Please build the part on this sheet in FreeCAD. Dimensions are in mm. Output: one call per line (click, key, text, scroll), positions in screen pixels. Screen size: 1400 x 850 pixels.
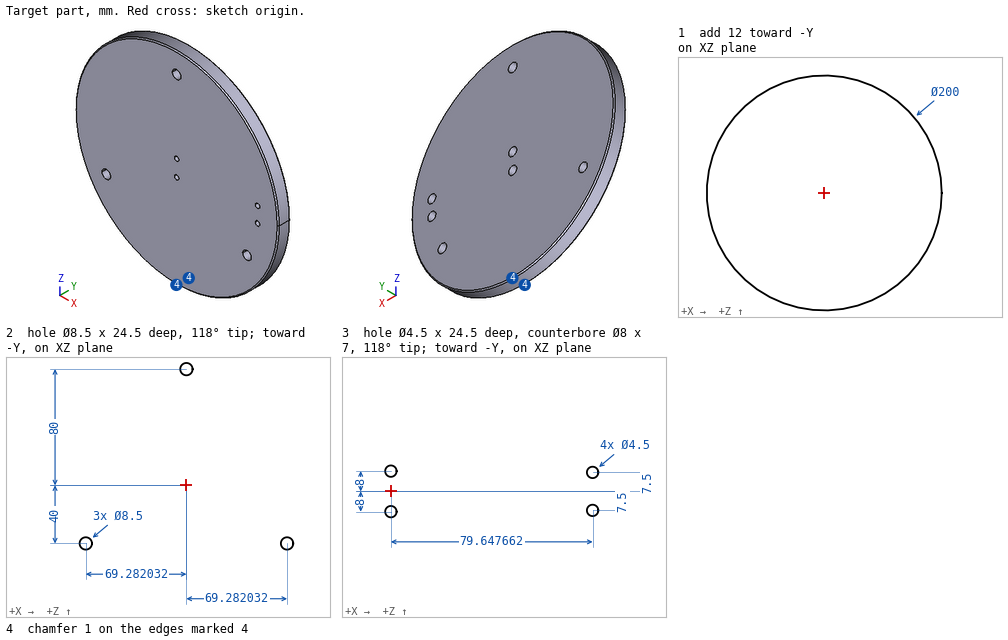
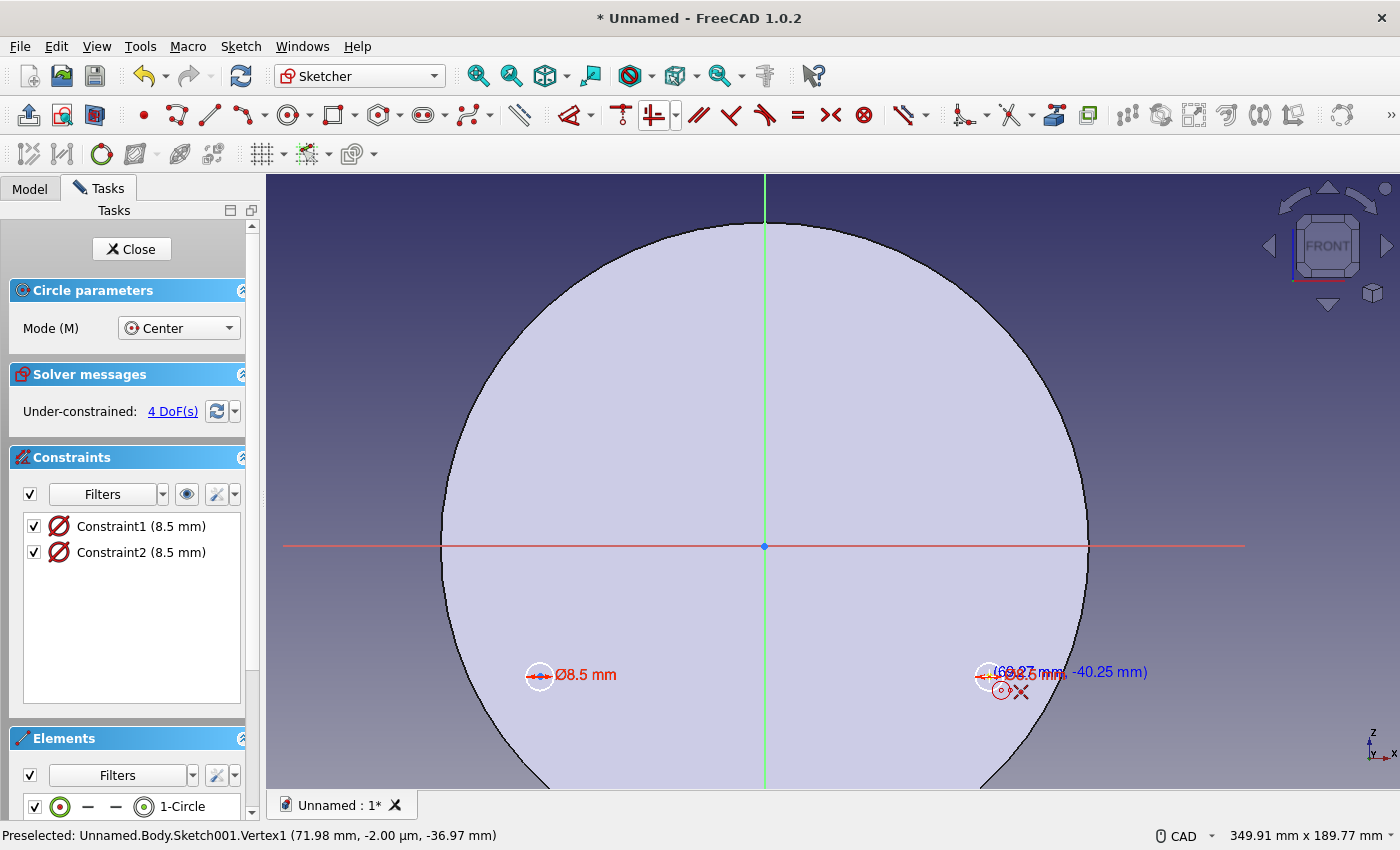
scroll(765, 287, up, 3)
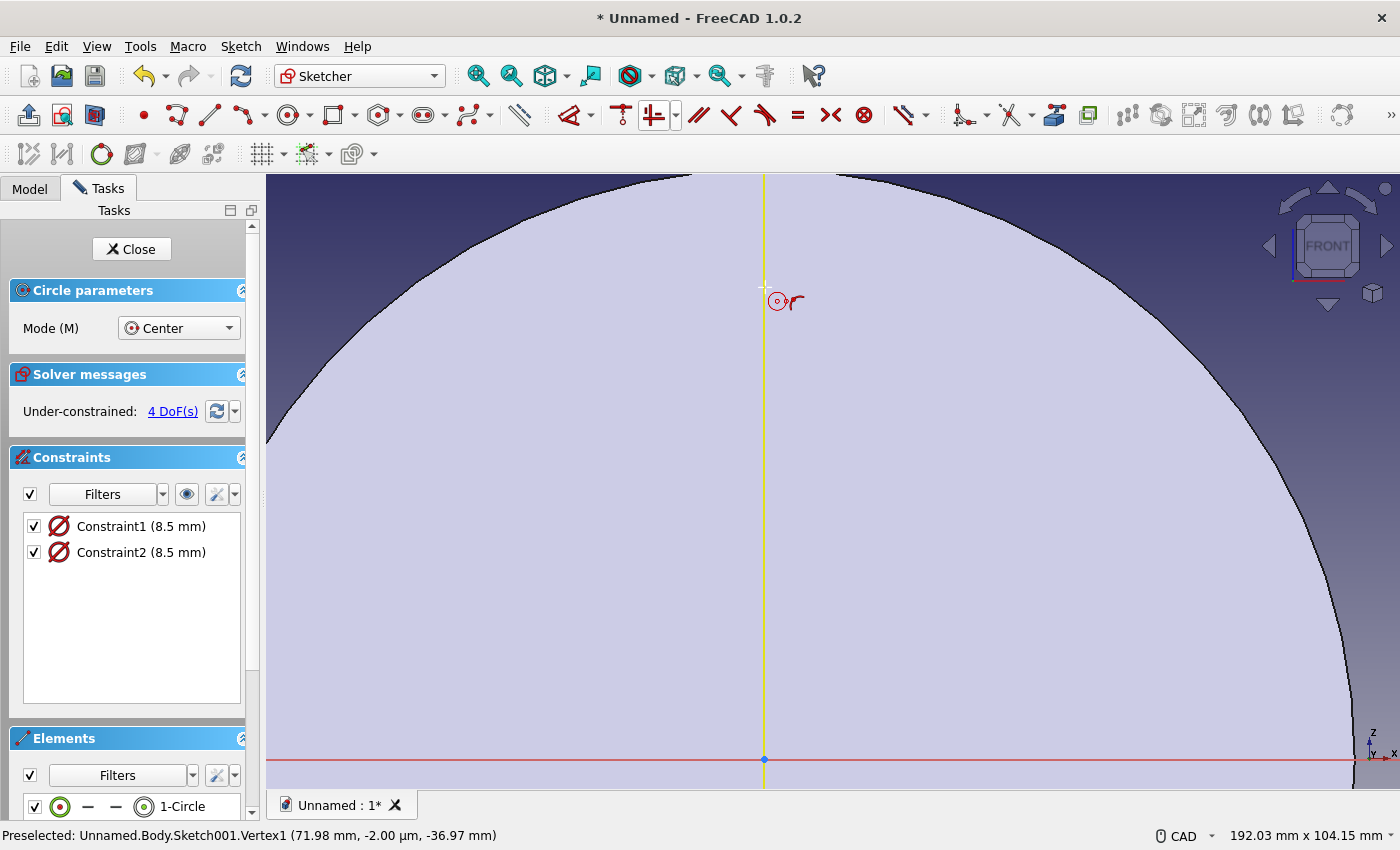
click(764, 287)
move(782, 270)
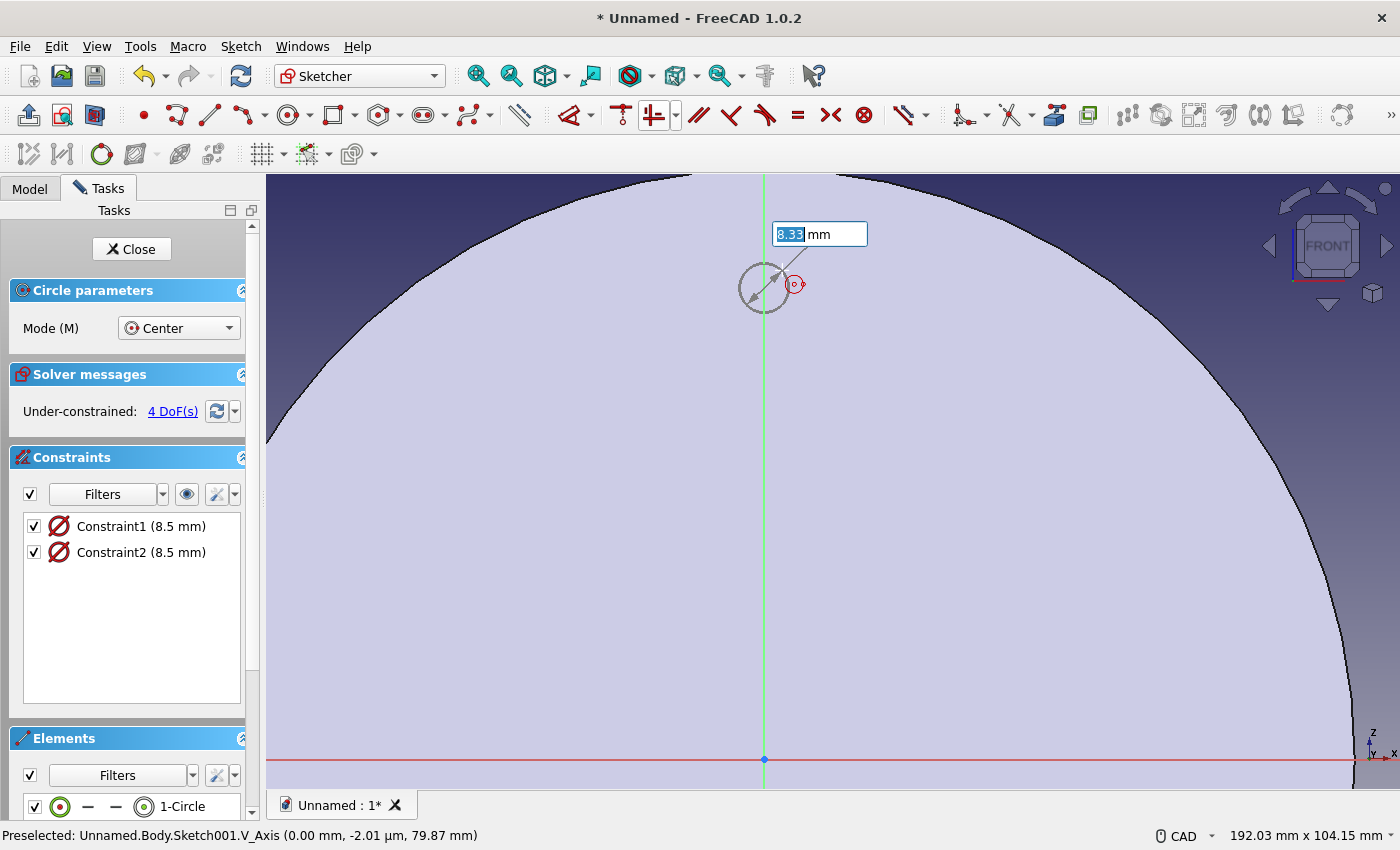
text(8.5)
key(Return)
key(Escape)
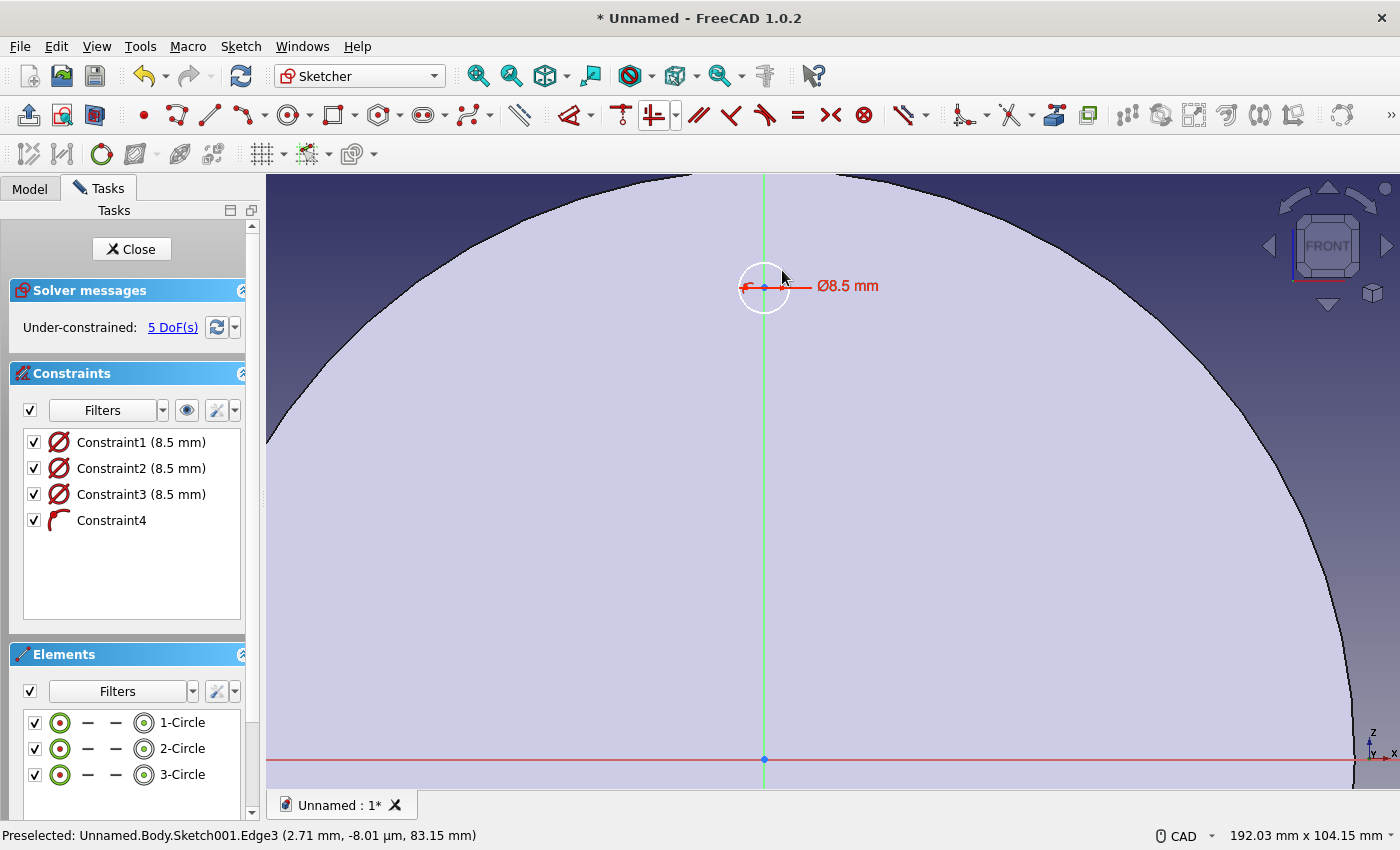
scroll(765, 287, down, 3)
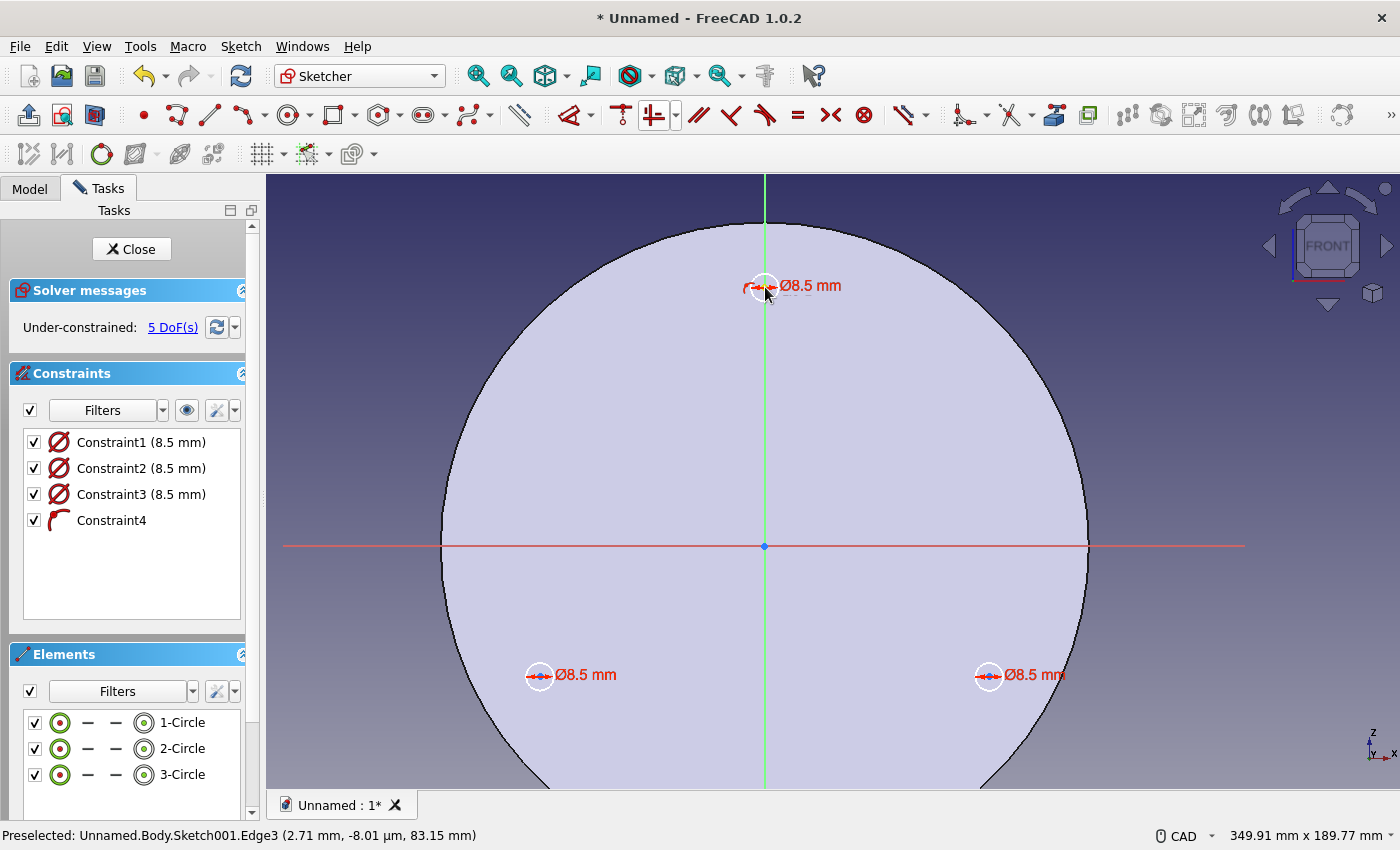
click(540, 677)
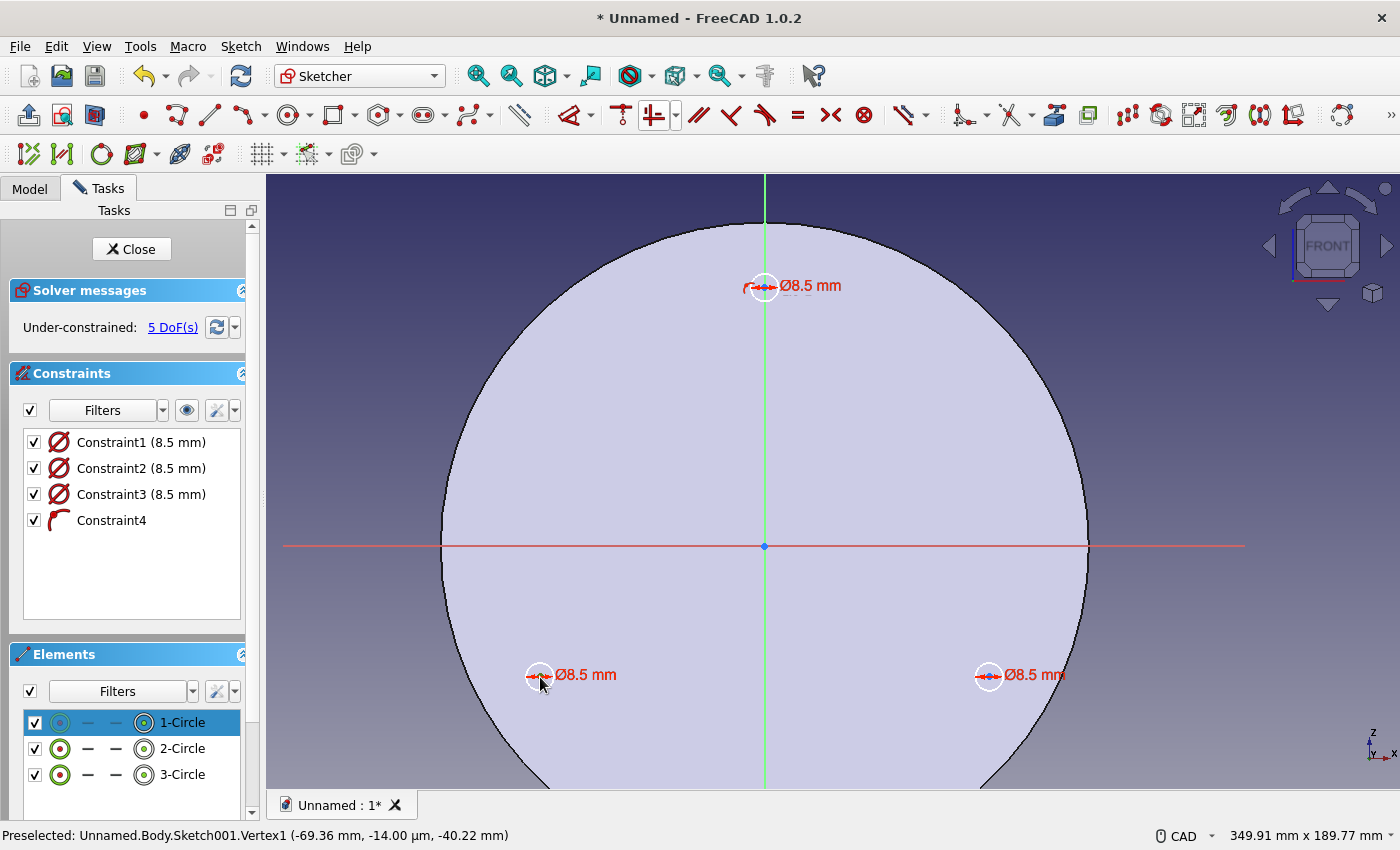
click(989, 677)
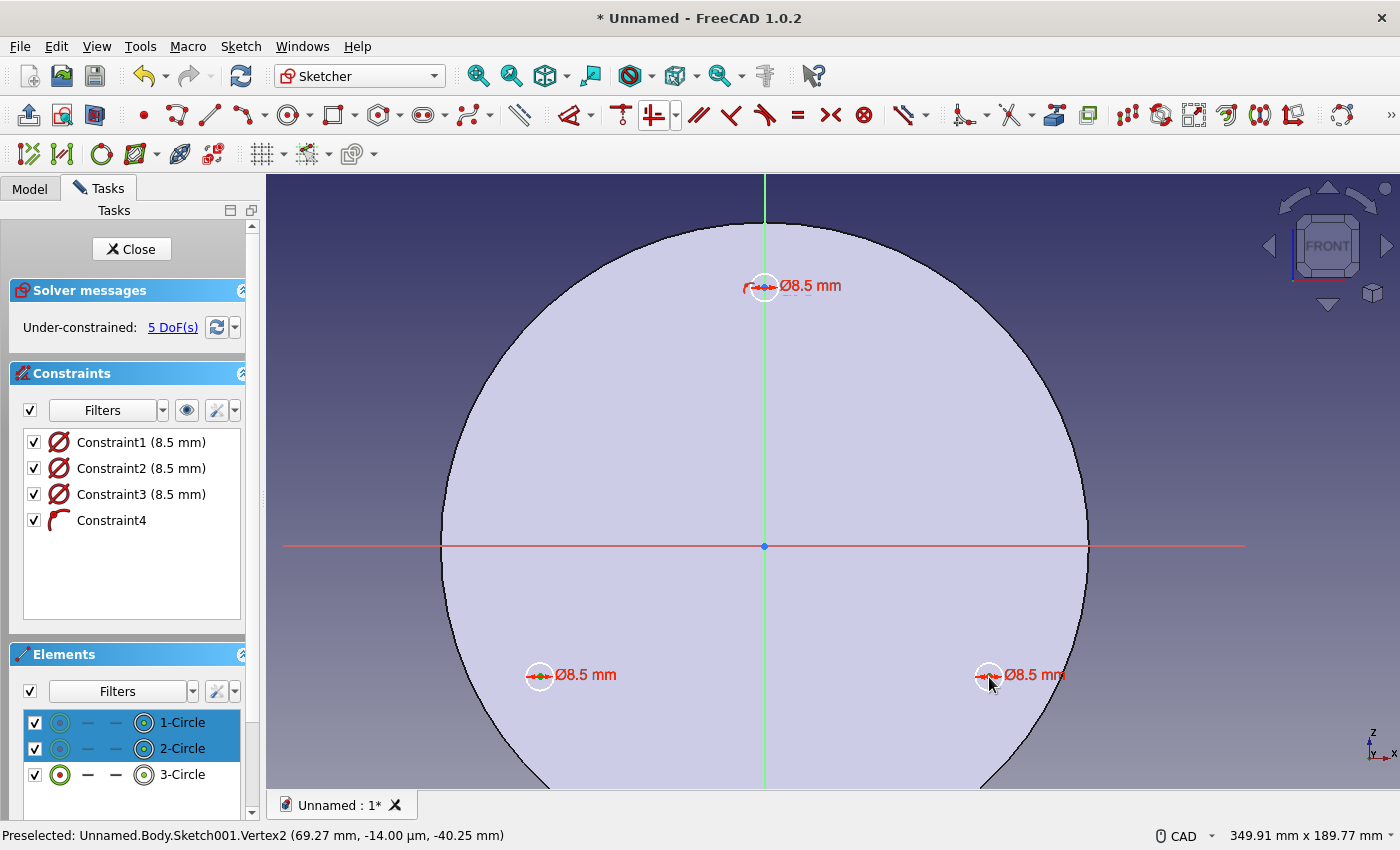
key(h)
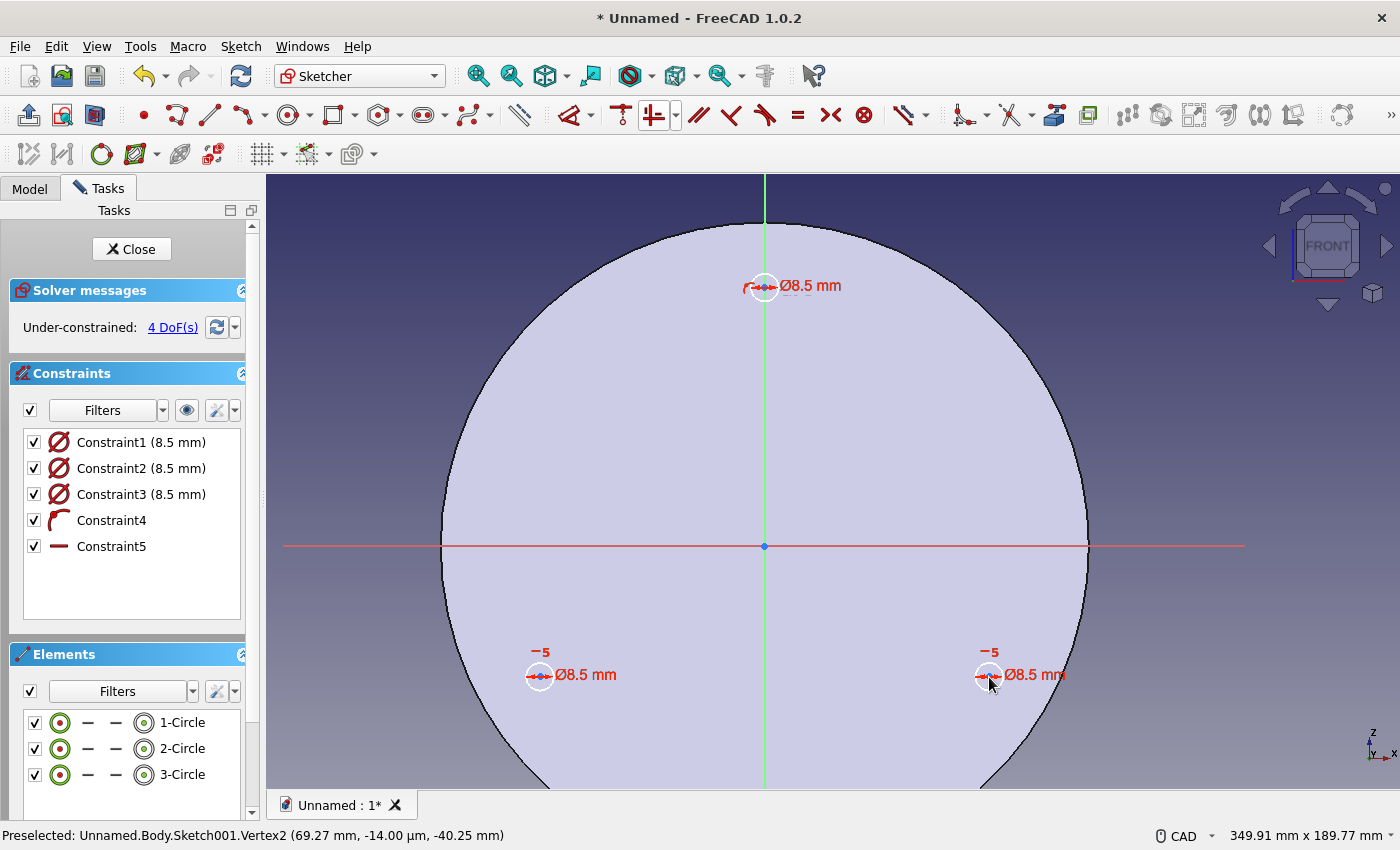
click(540, 677)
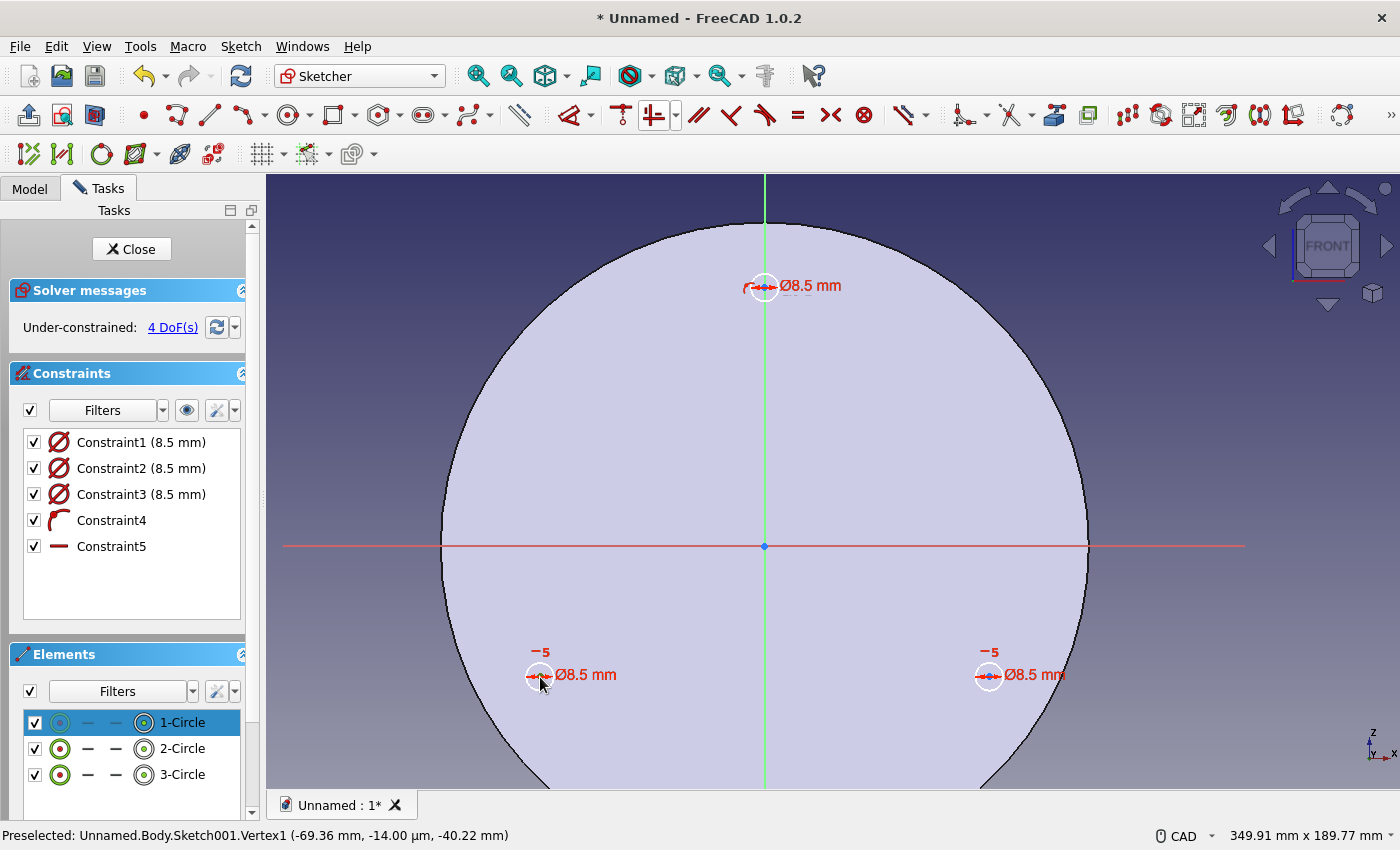
click(590, 116)